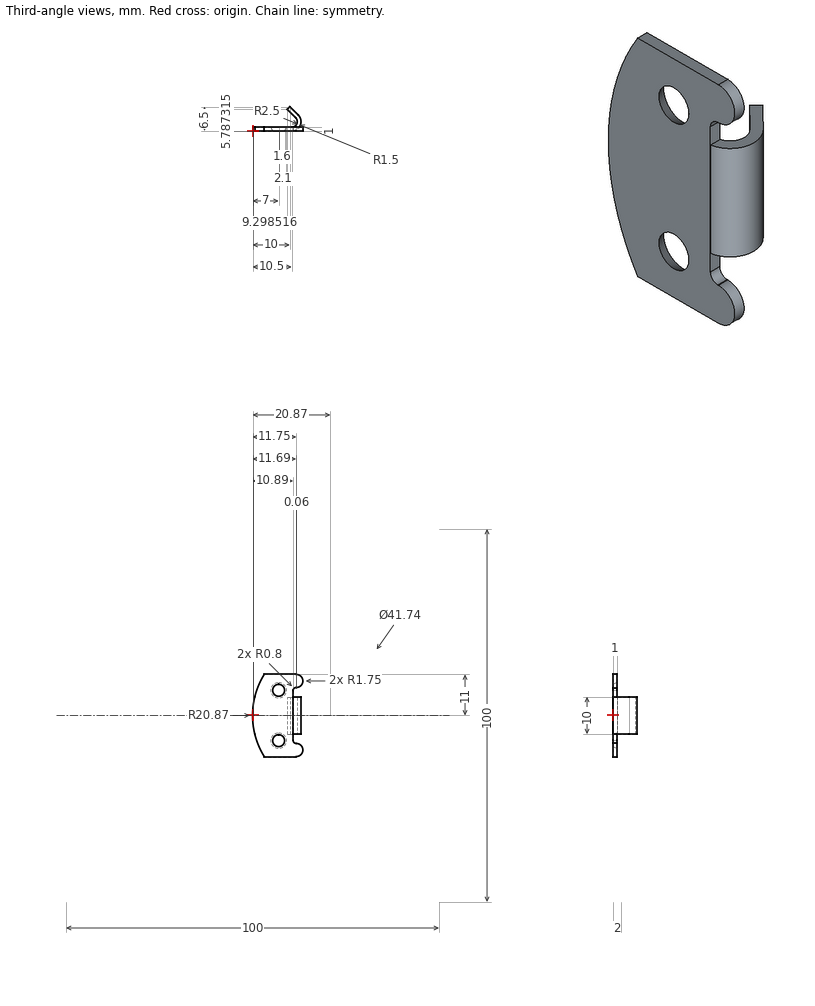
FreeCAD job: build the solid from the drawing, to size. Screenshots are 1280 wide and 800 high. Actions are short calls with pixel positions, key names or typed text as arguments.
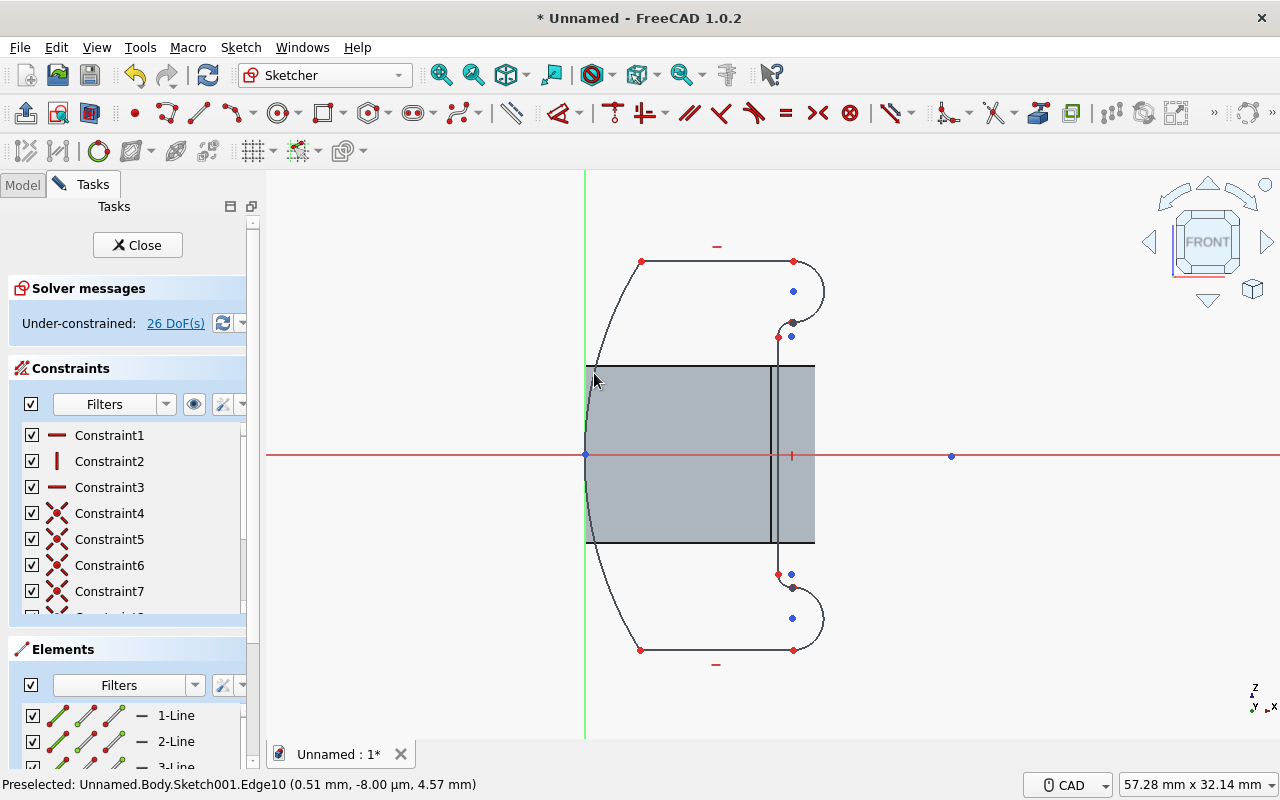
click(687, 261)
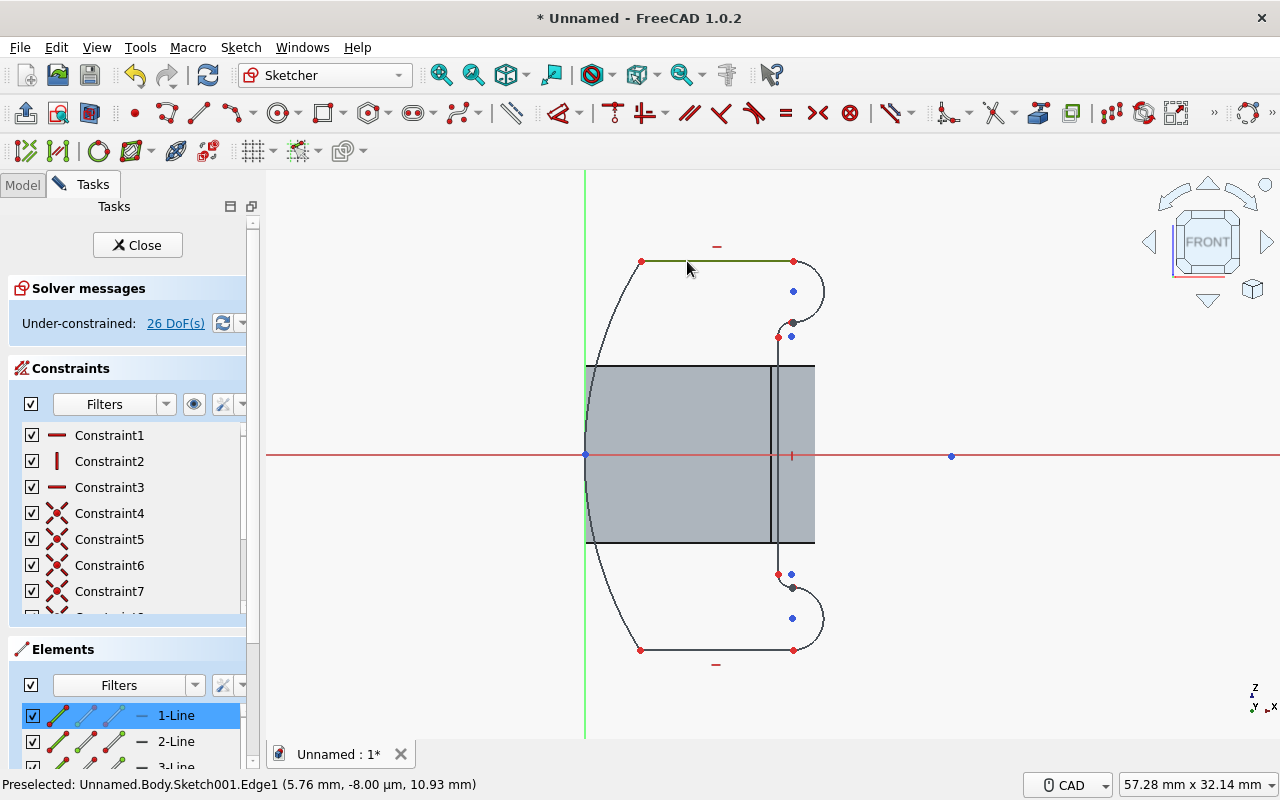
click(818, 310)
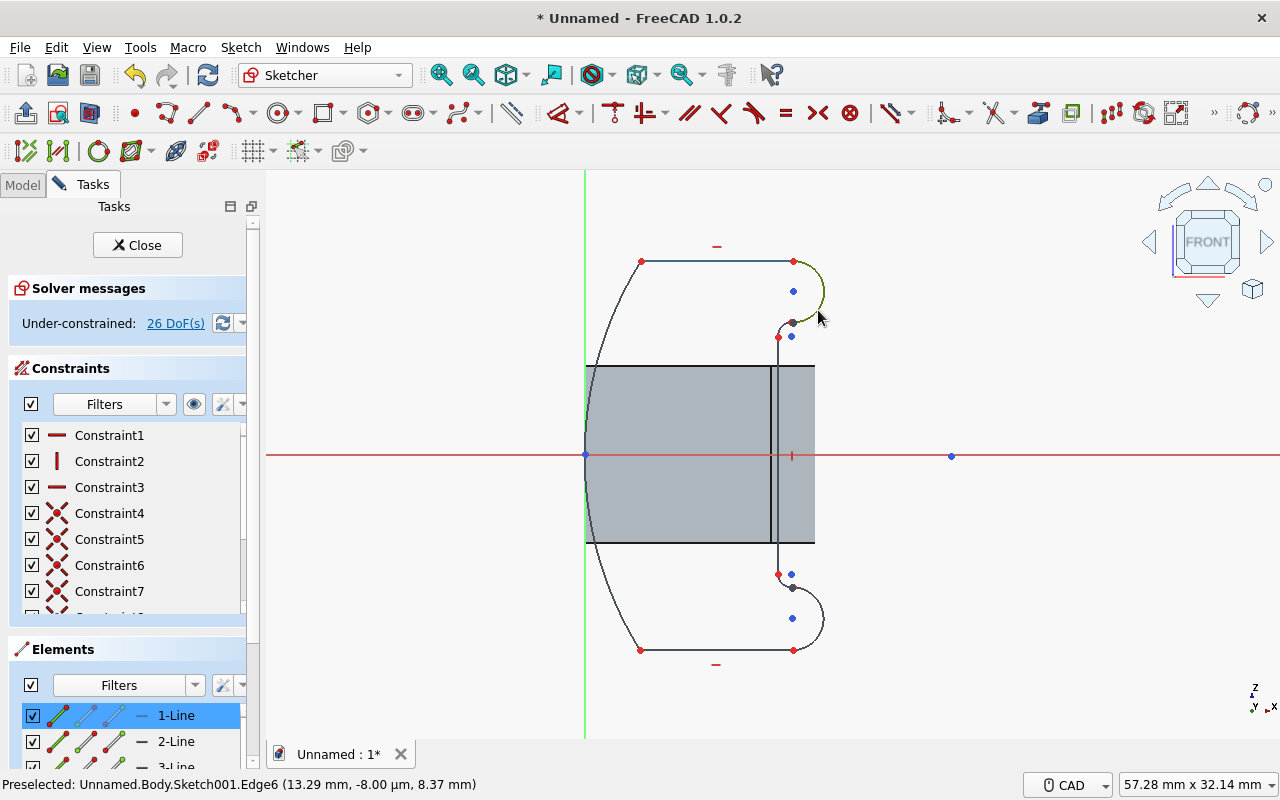
click(754, 114)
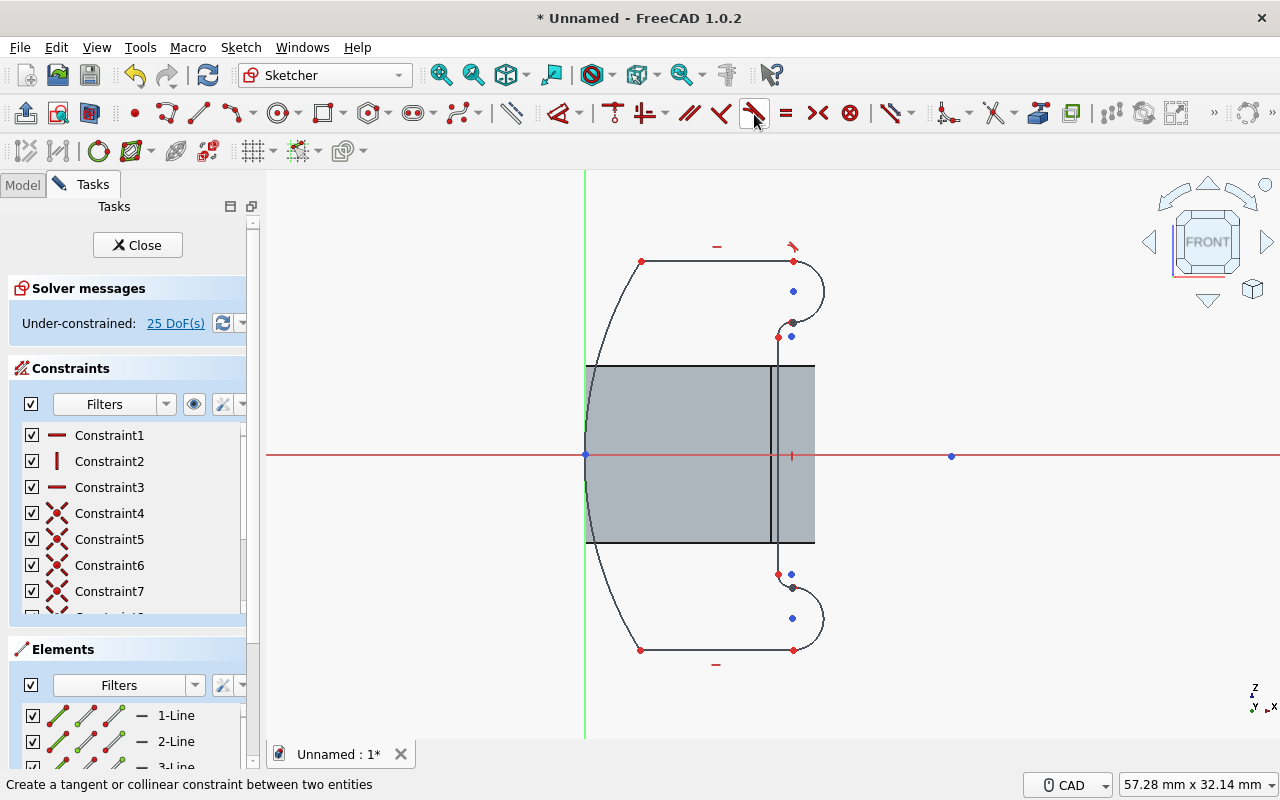
scroll(792, 323, up, 14)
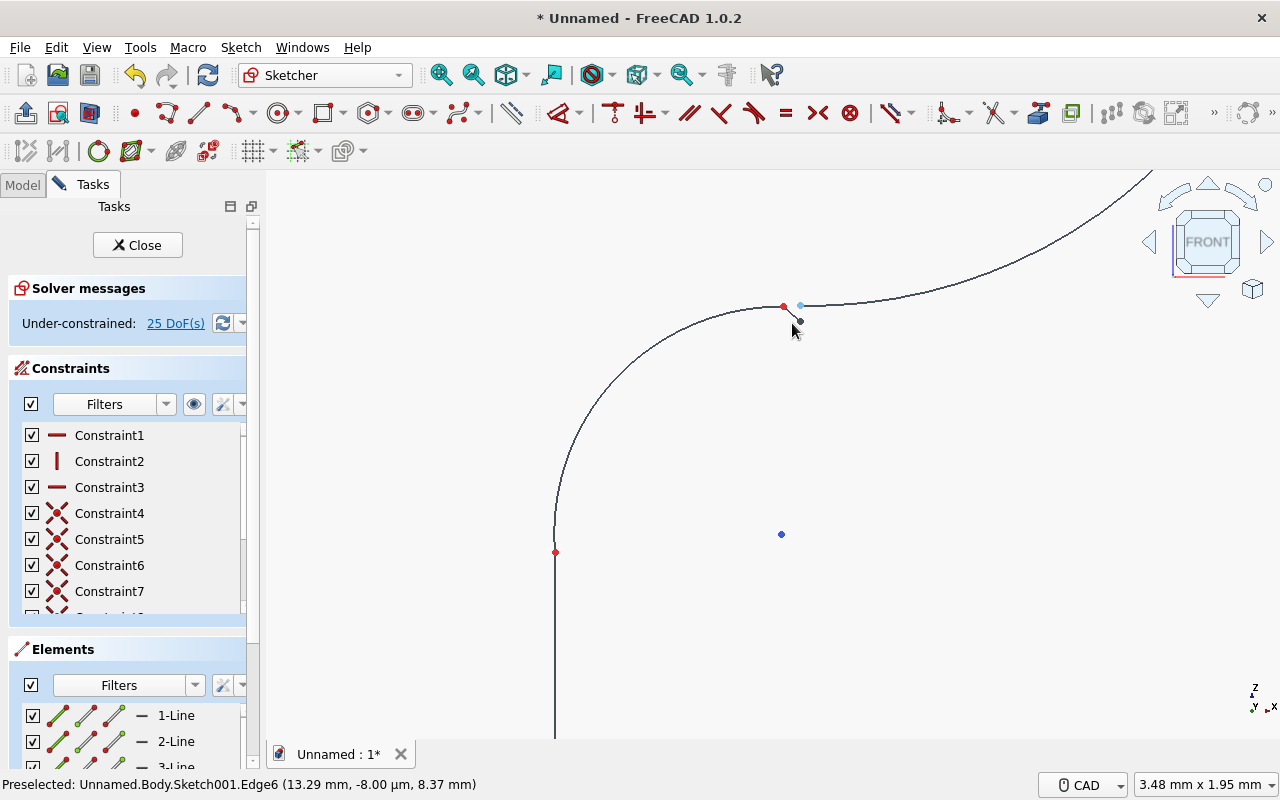
click(792, 314)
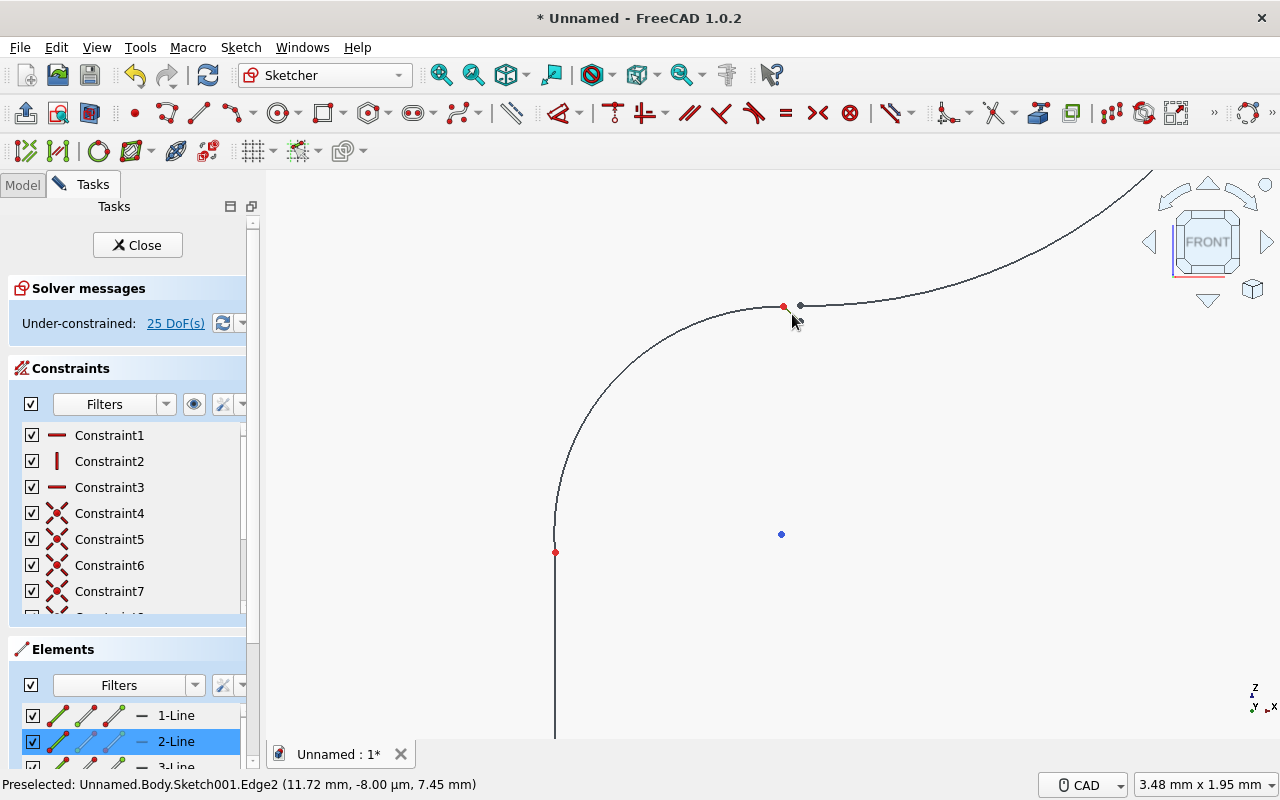
scroll(792, 323, down, 14)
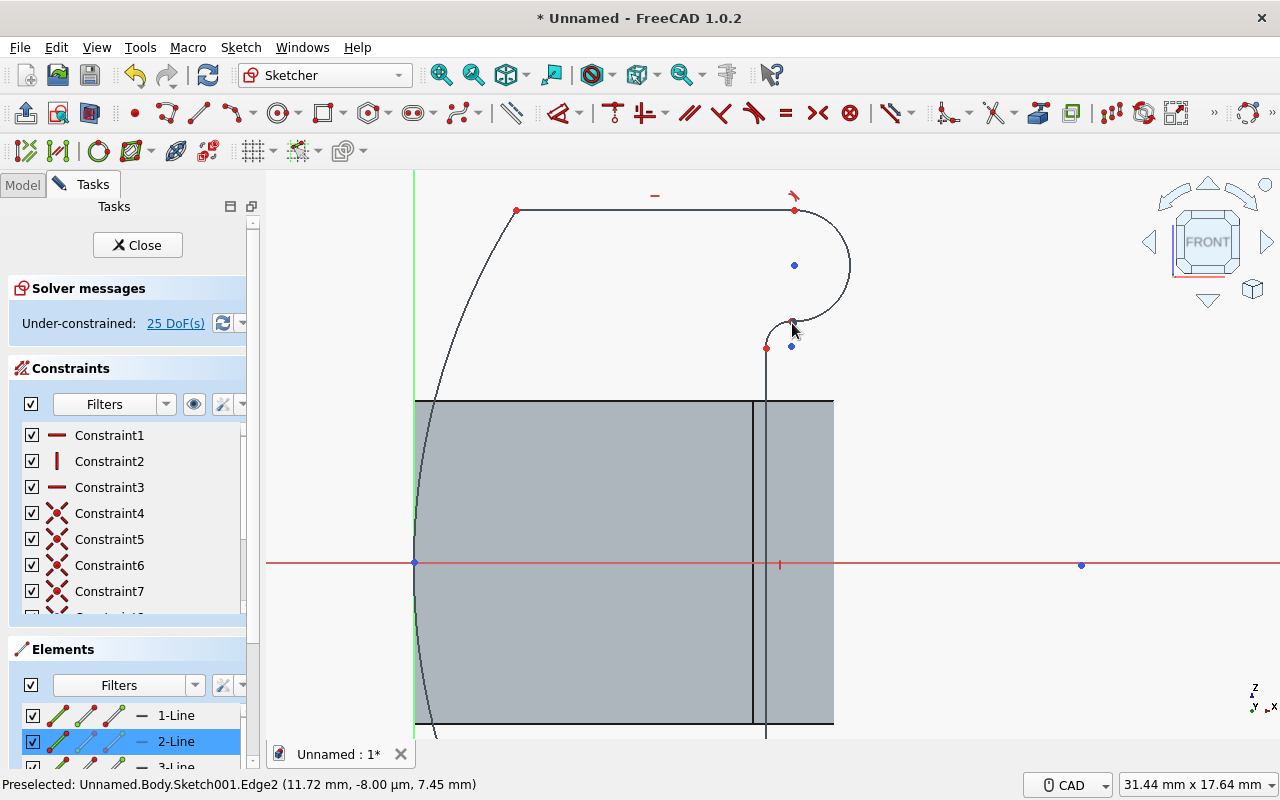
click(811, 317)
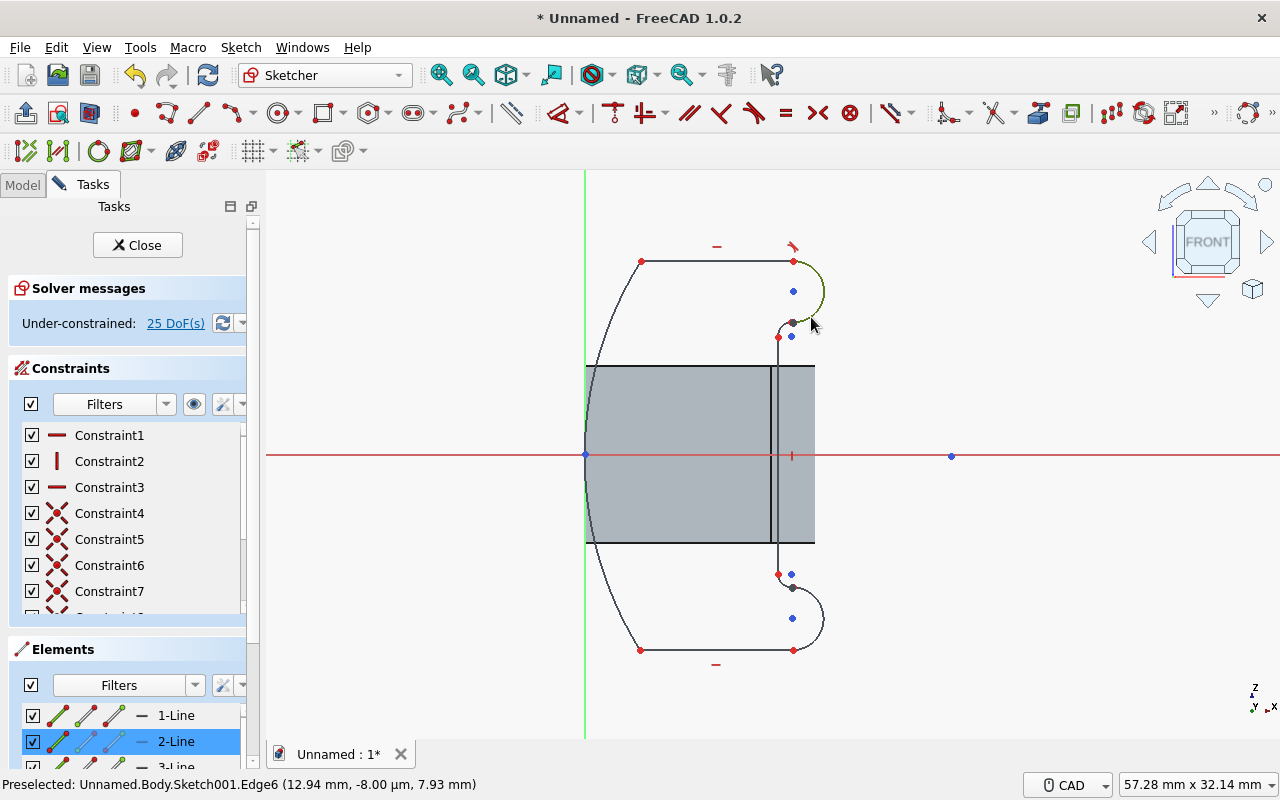
click(754, 114)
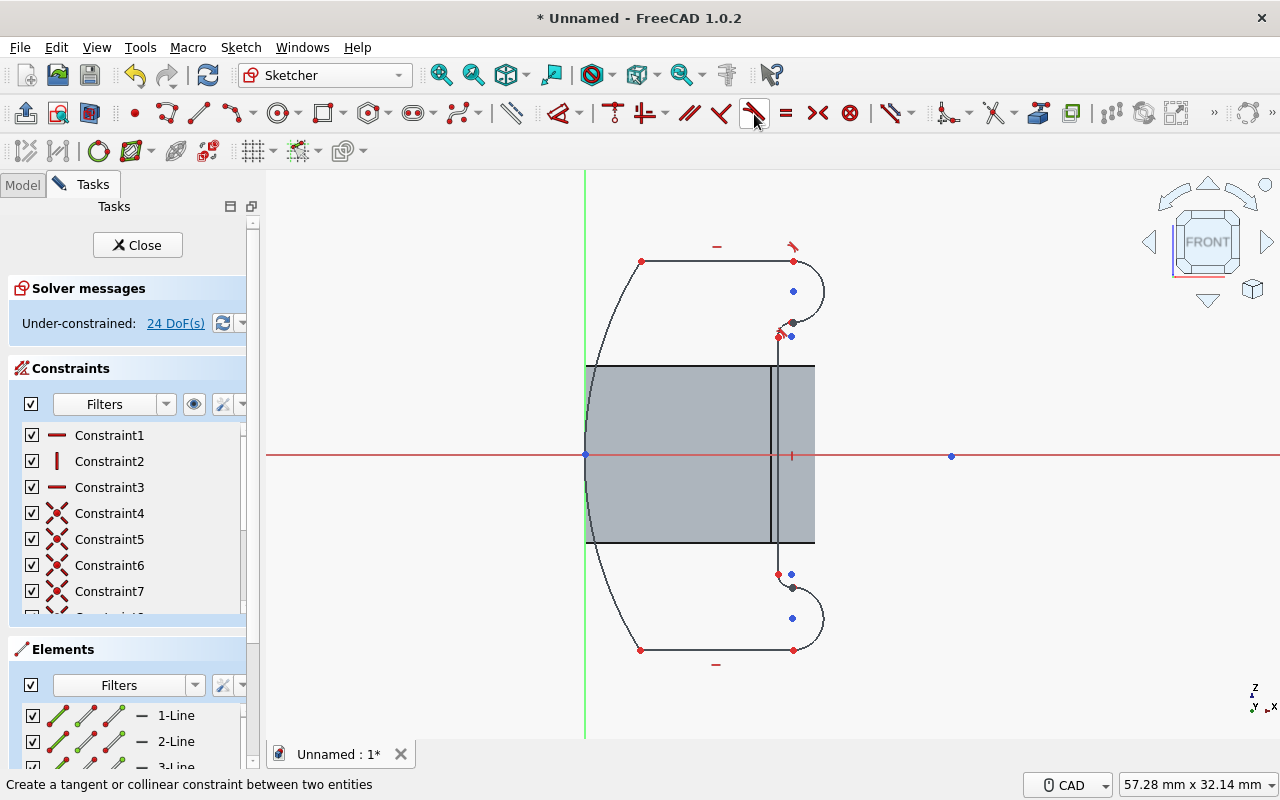
scroll(792, 323, up, 14)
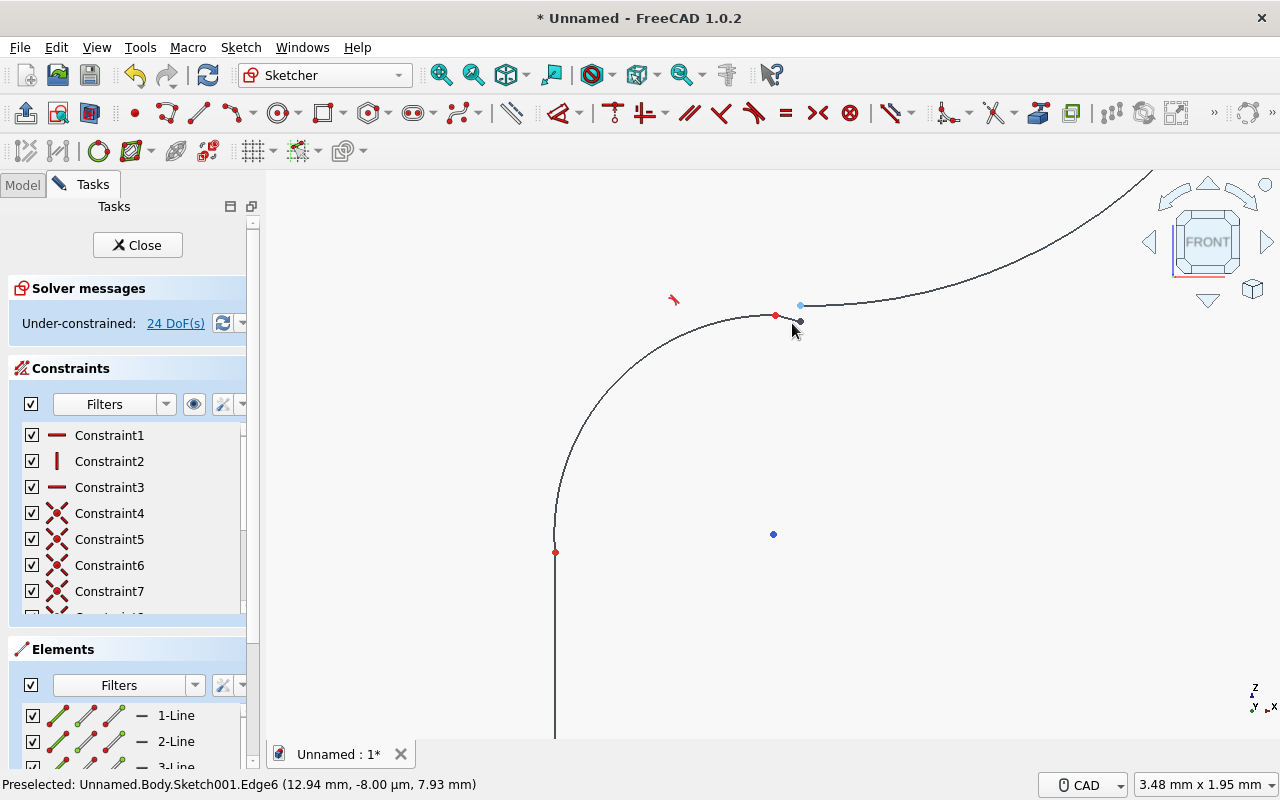
click(788, 319)